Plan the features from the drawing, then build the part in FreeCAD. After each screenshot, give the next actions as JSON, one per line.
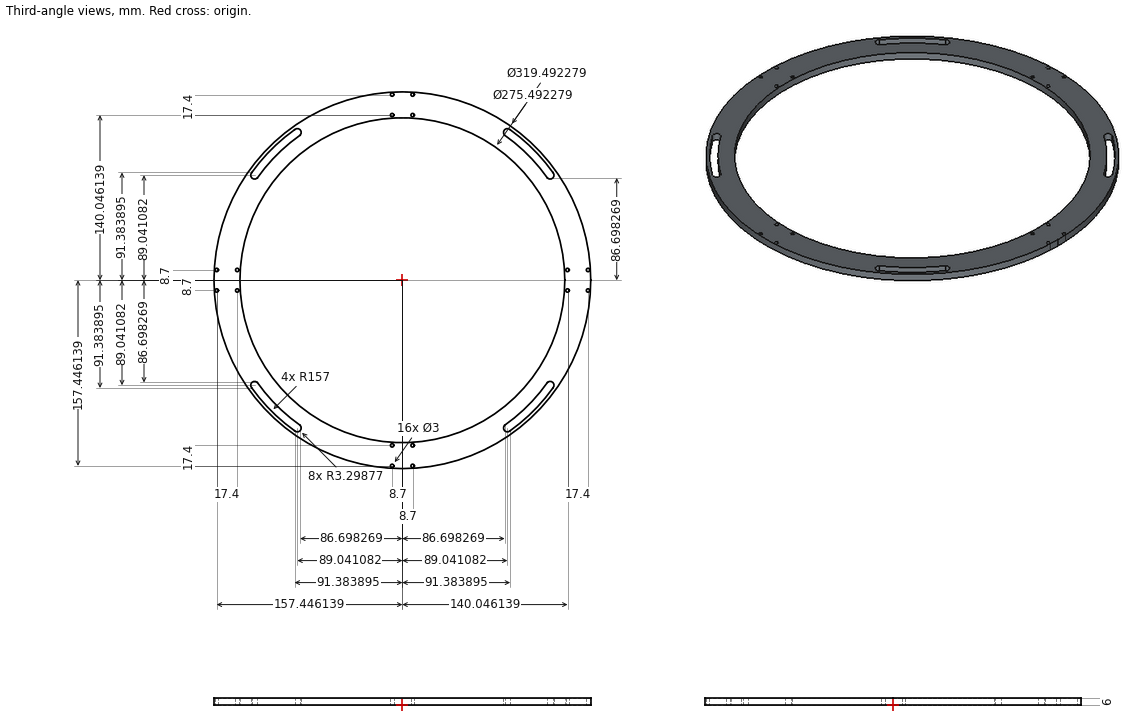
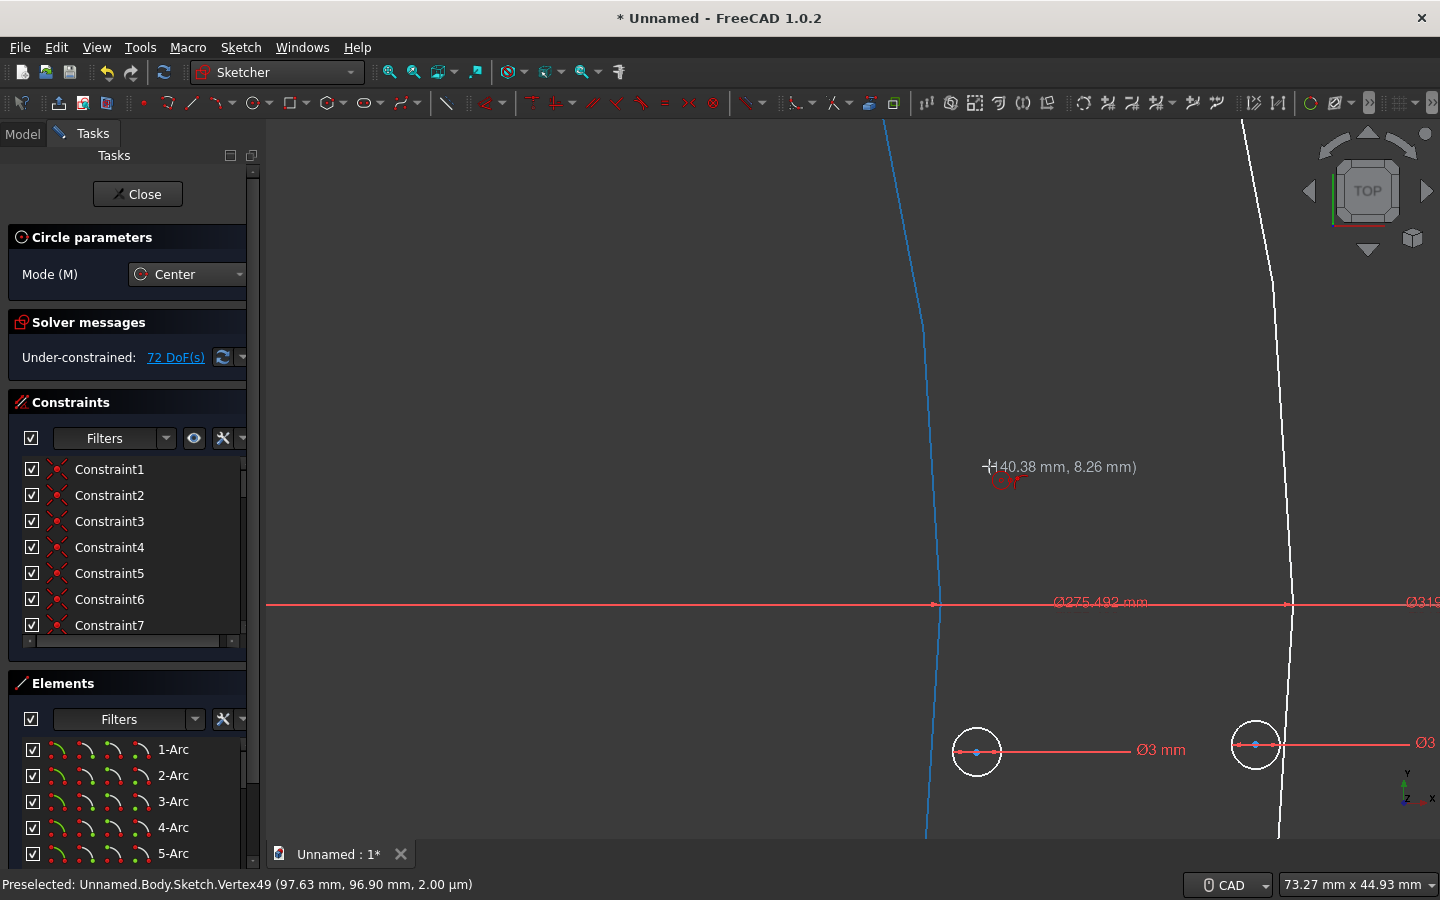
{"action": "left_click", "coordinate": [978, 465]}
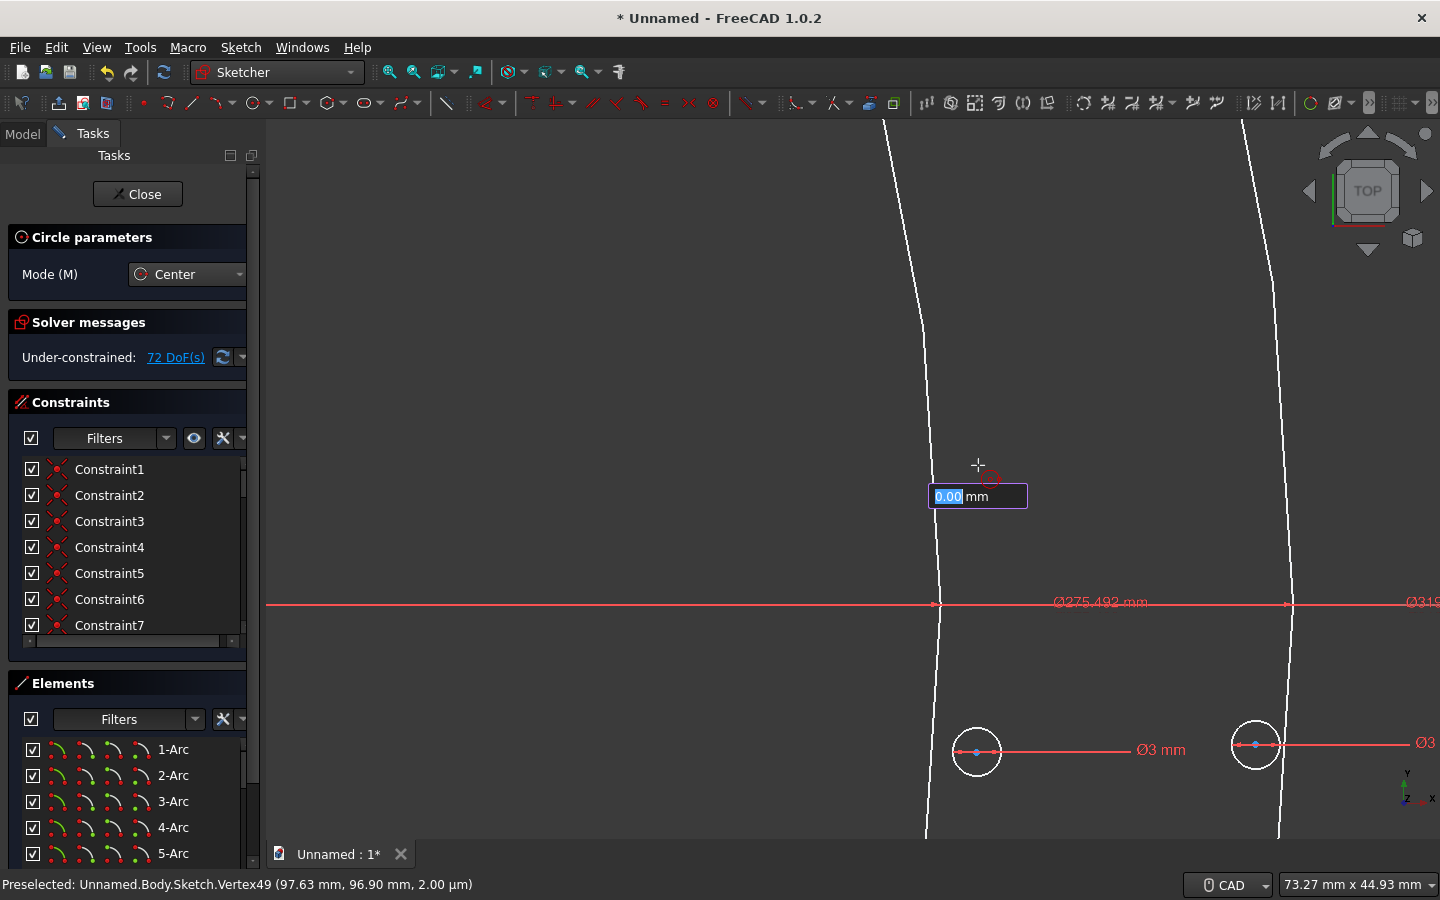
{"action": "scroll", "coordinate": [989, 466], "scroll_direction": "down", "scroll_amount": 12}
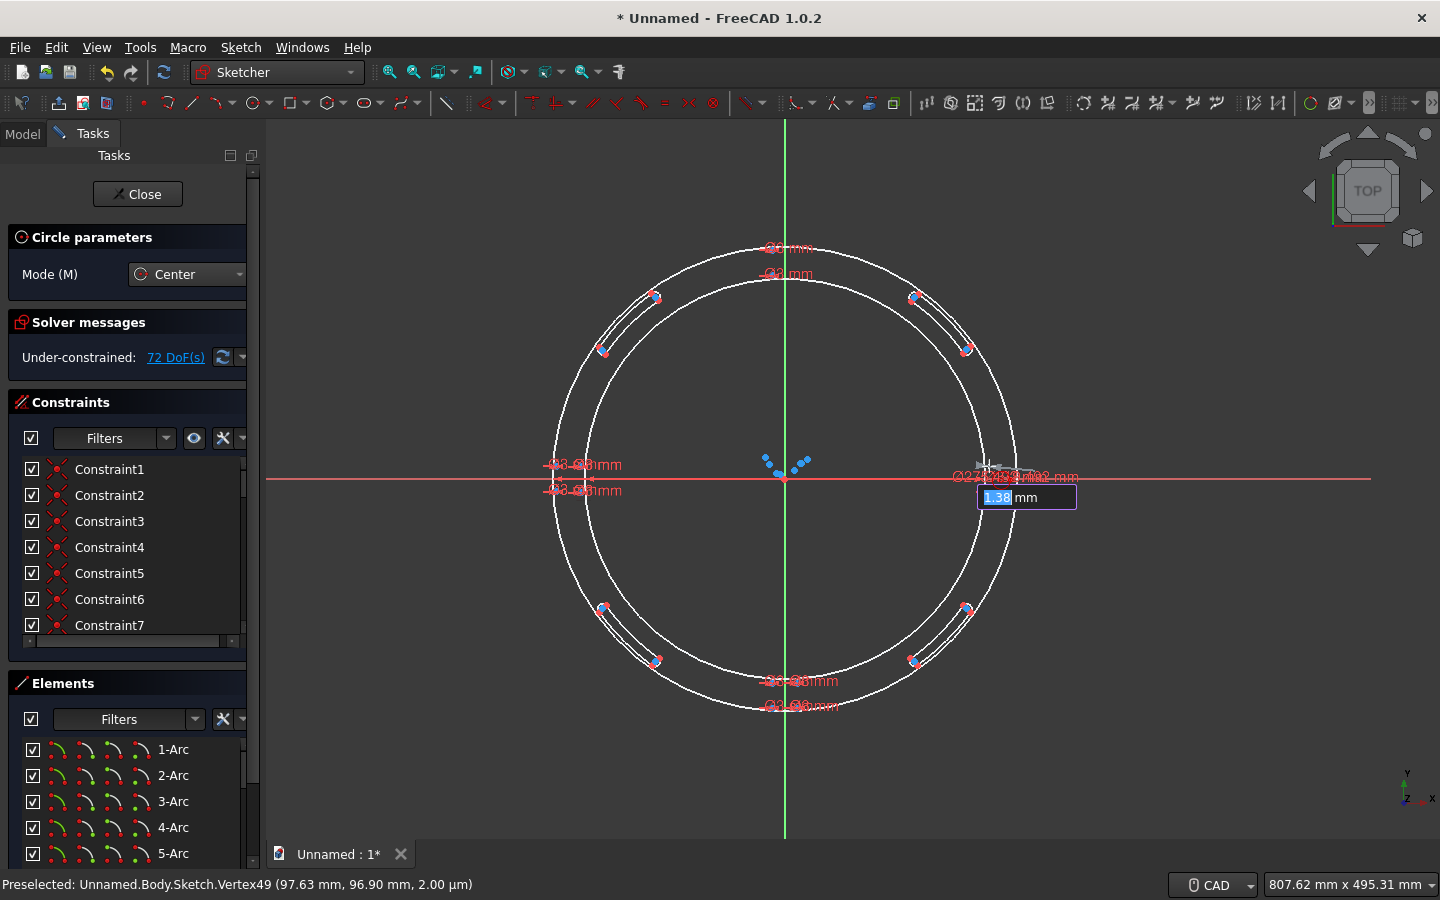
{"action": "scroll", "coordinate": [990, 465], "scroll_direction": "up", "scroll_amount": 6}
{"action": "mouse_move", "coordinate": [989, 463]}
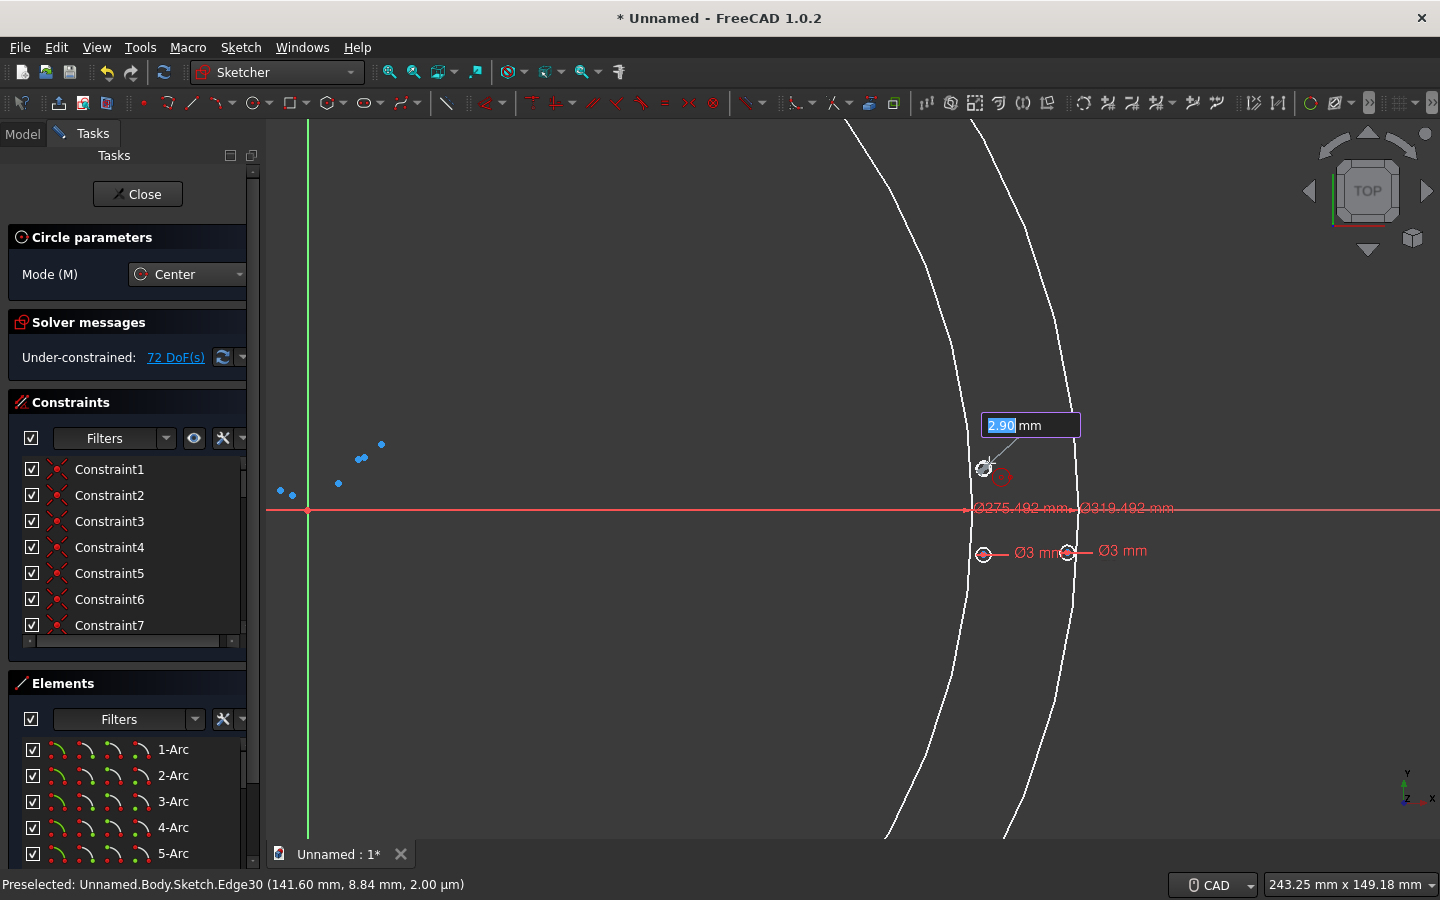
{"action": "type", "text": "3"}
{"action": "key", "text": "Return"}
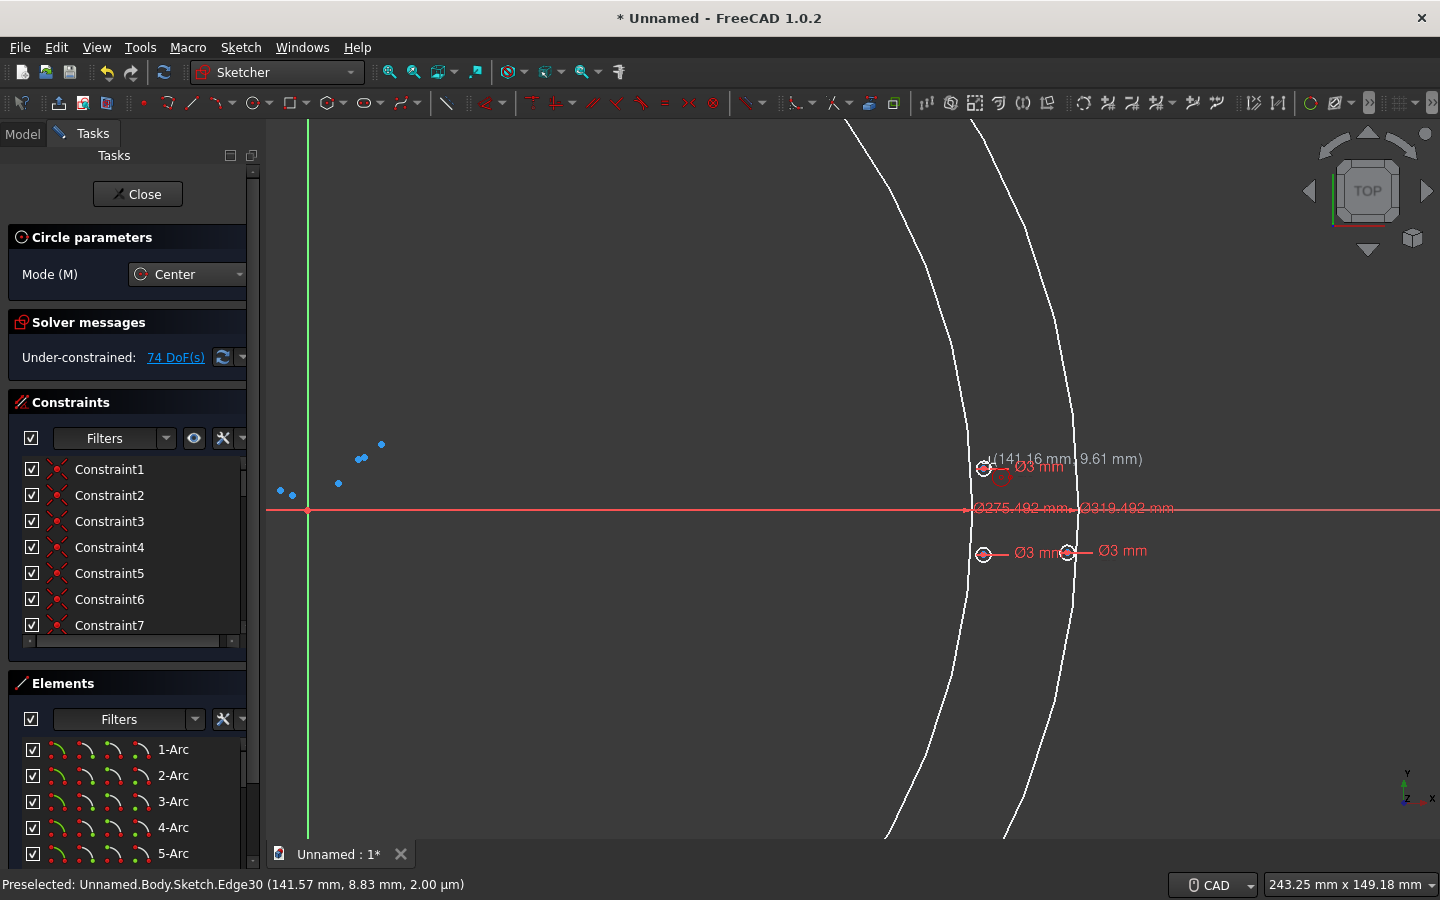
{"action": "scroll", "coordinate": [1068, 468], "scroll_direction": "up", "scroll_amount": 6}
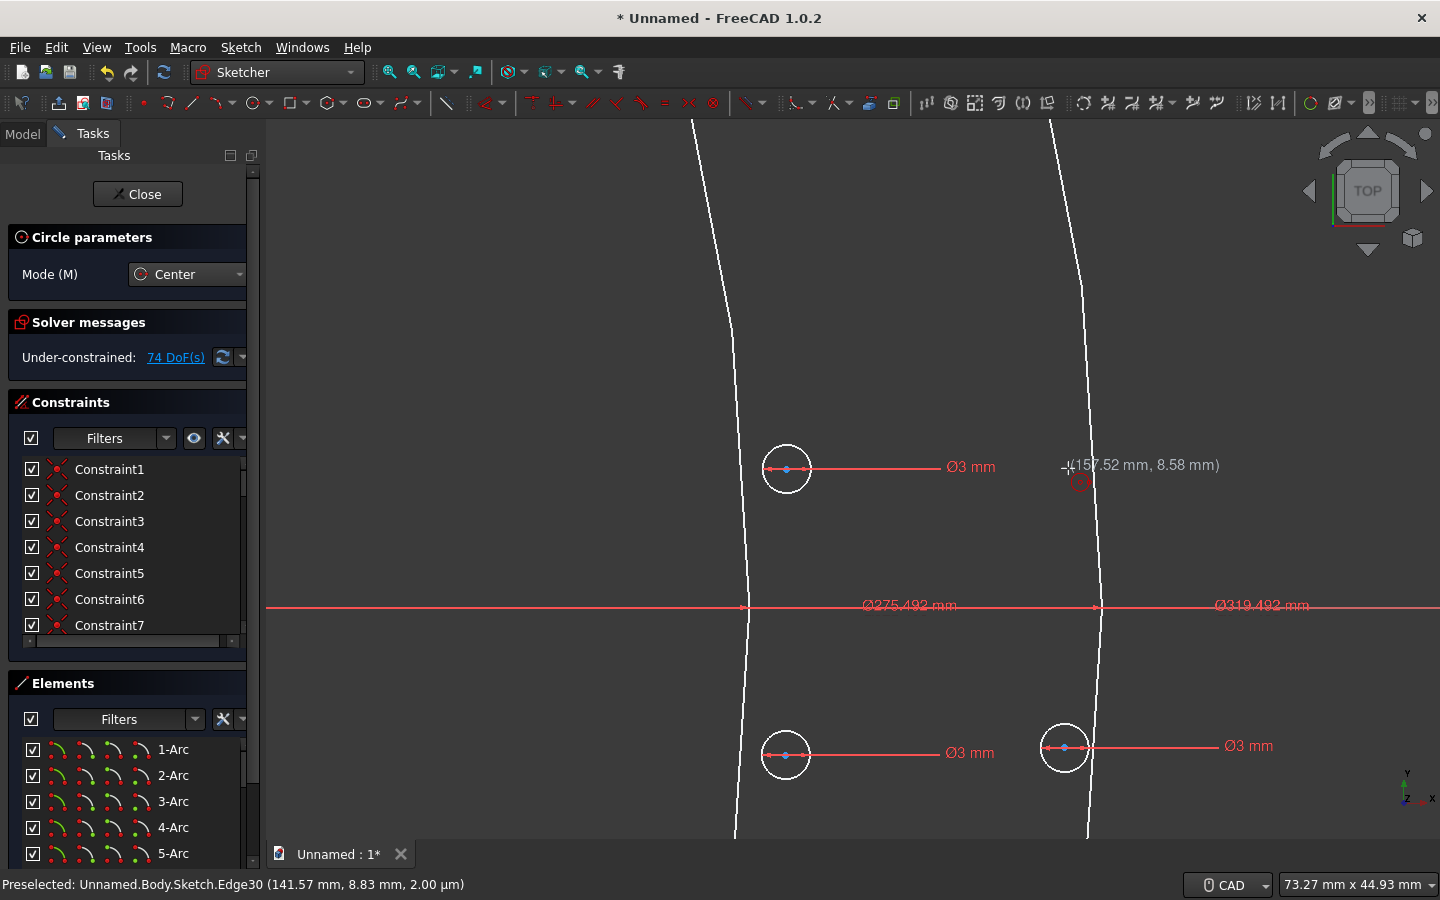
{"action": "left_click", "coordinate": [1065, 468]}
{"action": "mouse_move", "coordinate": [1082, 451]}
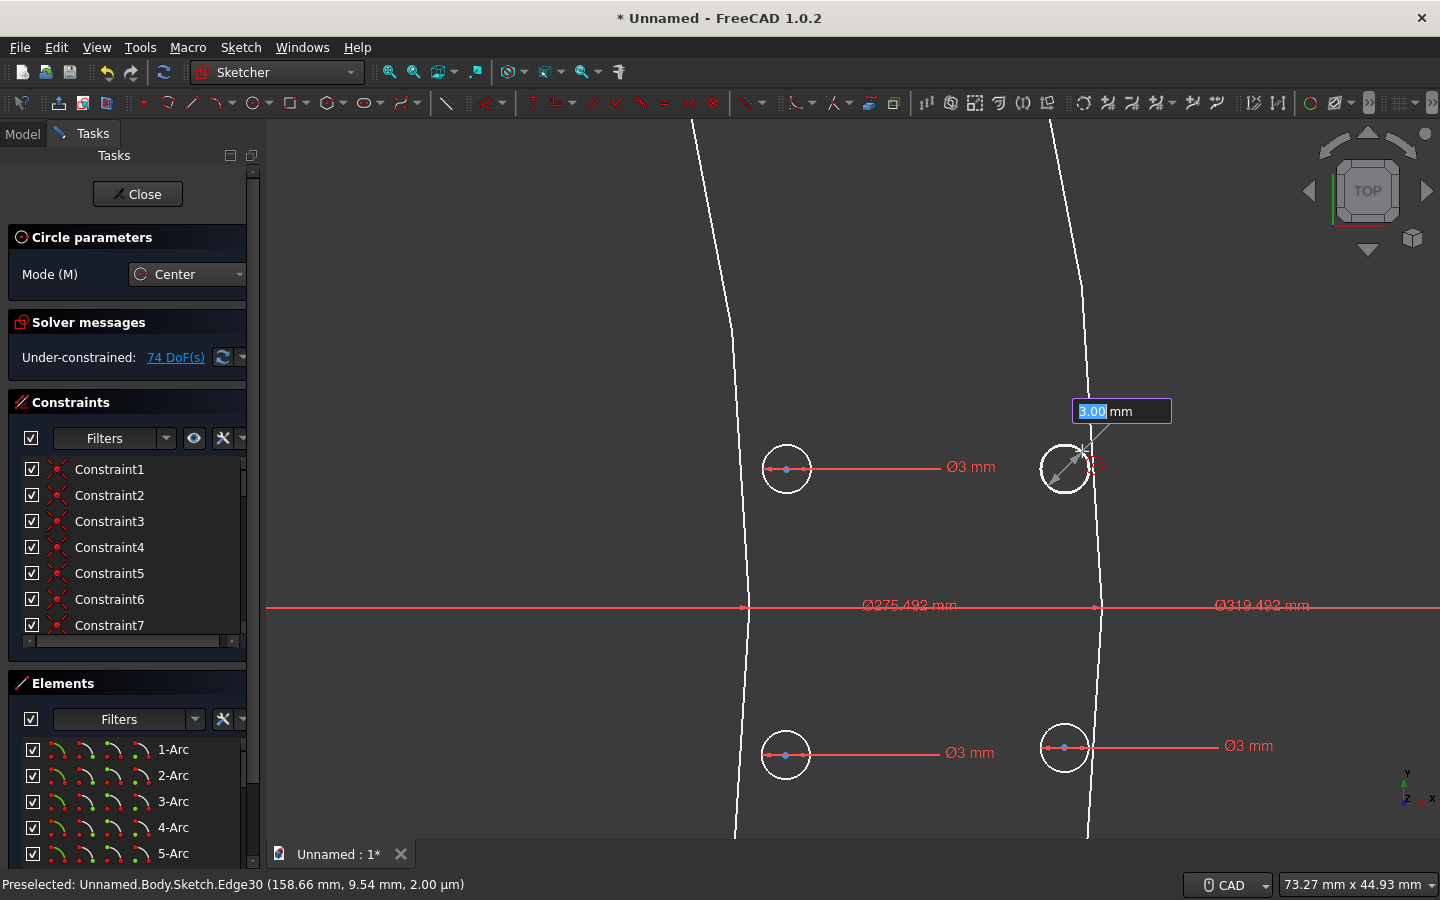
{"action": "type", "text": "3"}
{"action": "key", "text": "Return"}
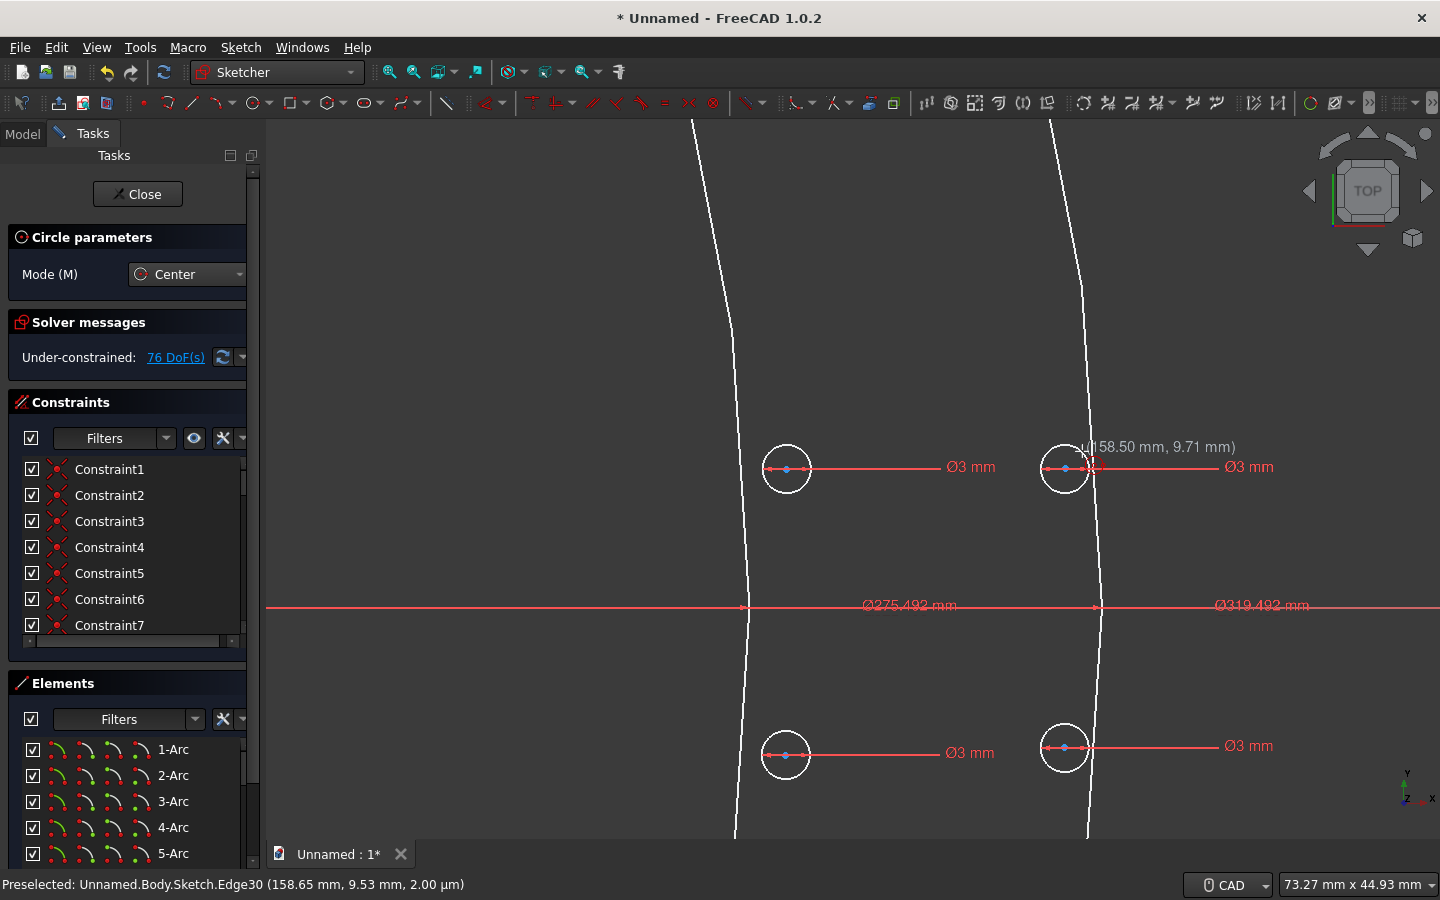
{"action": "scroll", "coordinate": [1008, 466], "scroll_direction": "down", "scroll_amount": 12}